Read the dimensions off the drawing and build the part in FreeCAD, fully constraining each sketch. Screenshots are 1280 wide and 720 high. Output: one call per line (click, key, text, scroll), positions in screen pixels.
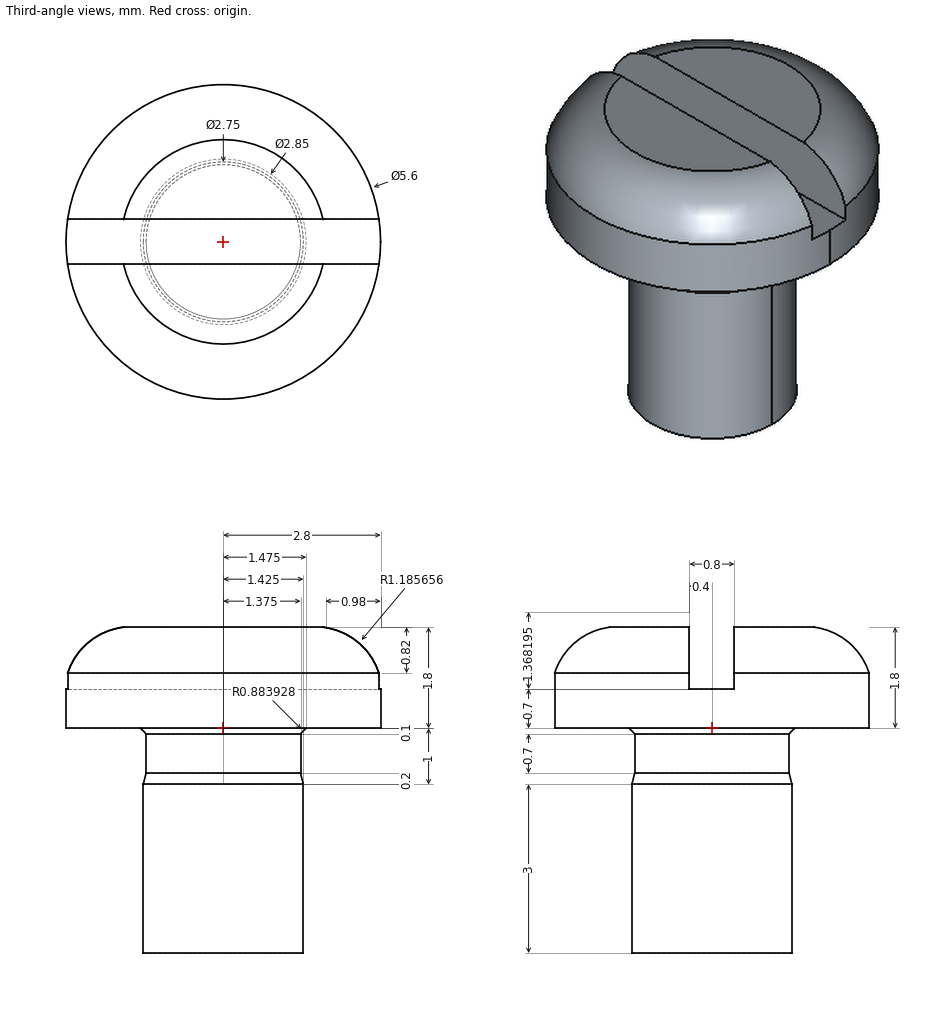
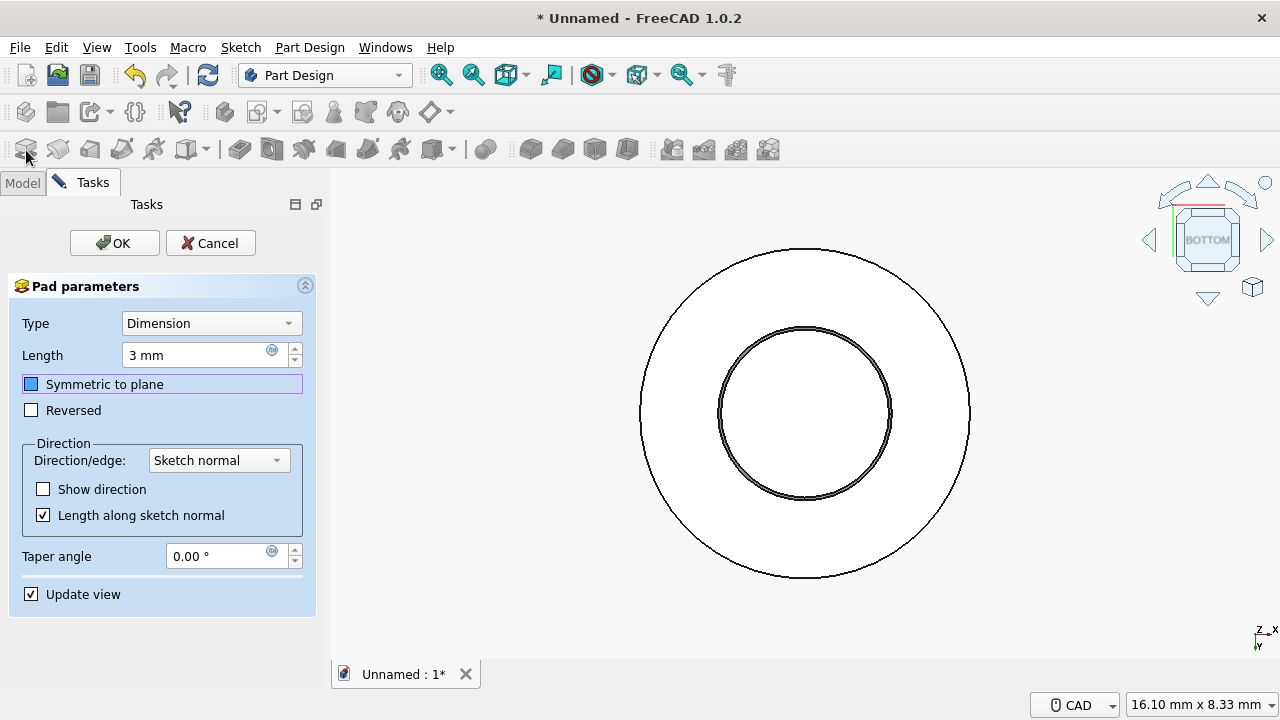
click(115, 243)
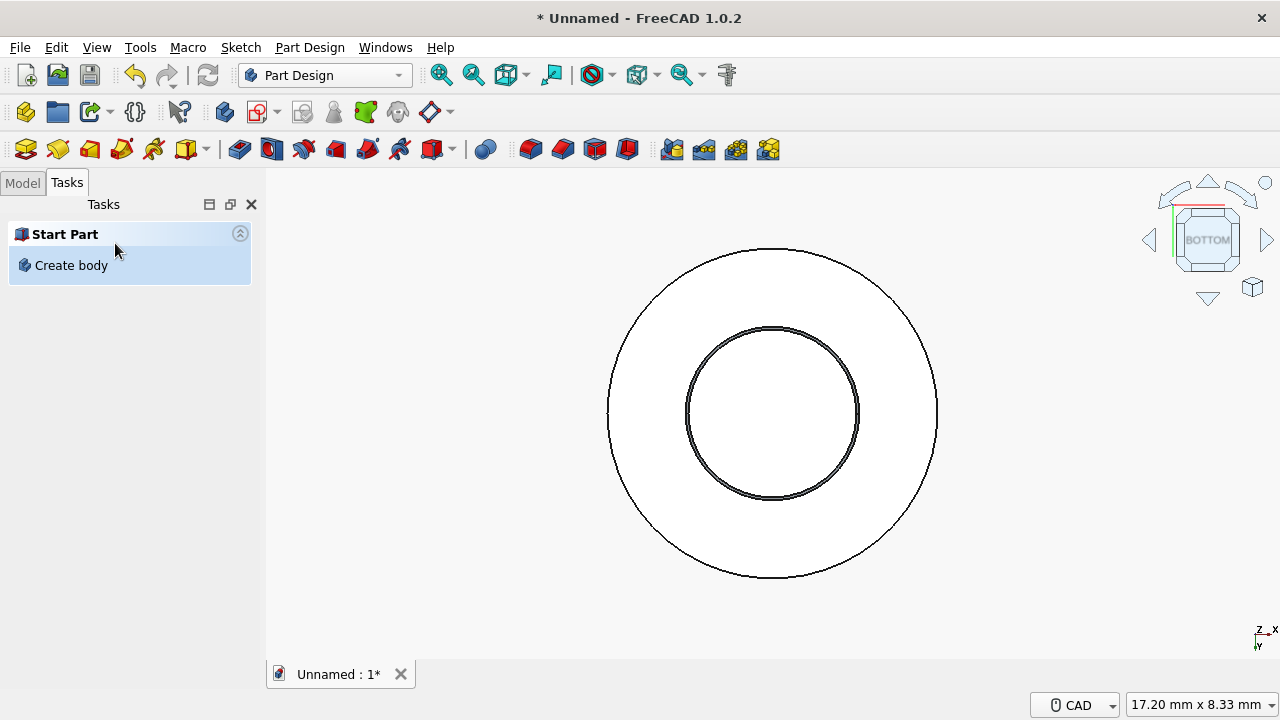
click(258, 112)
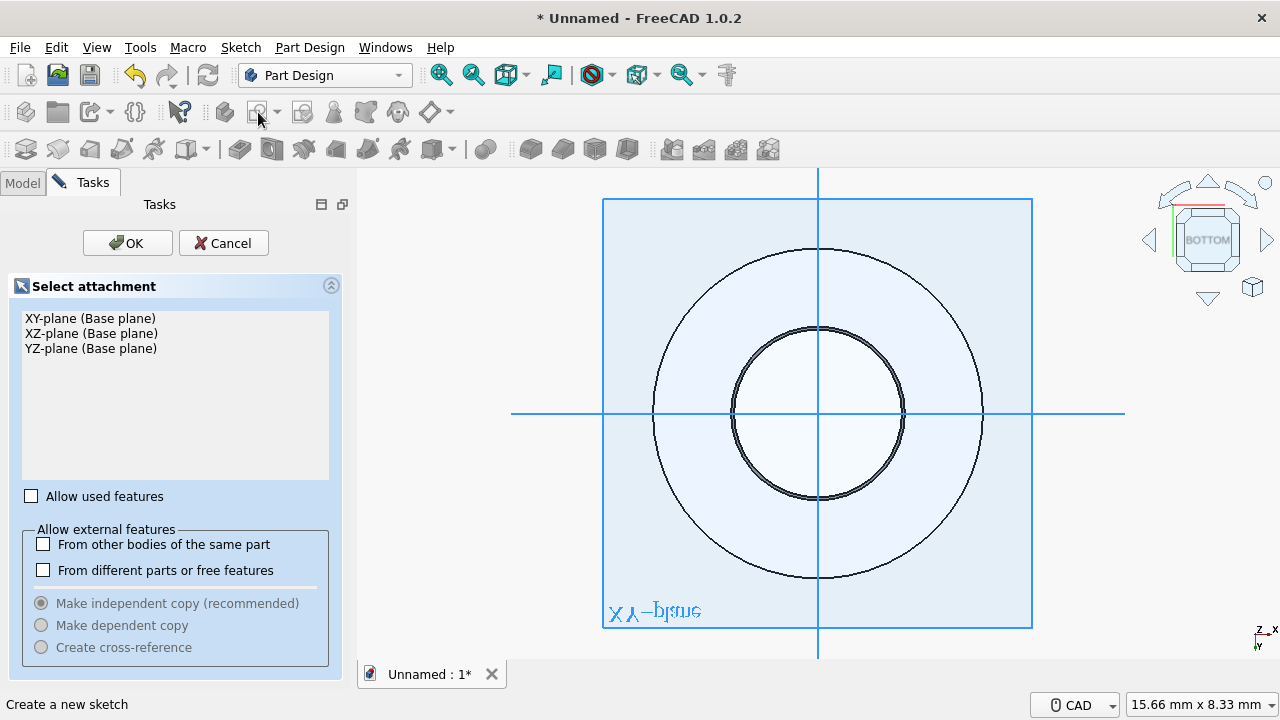
click(82, 334)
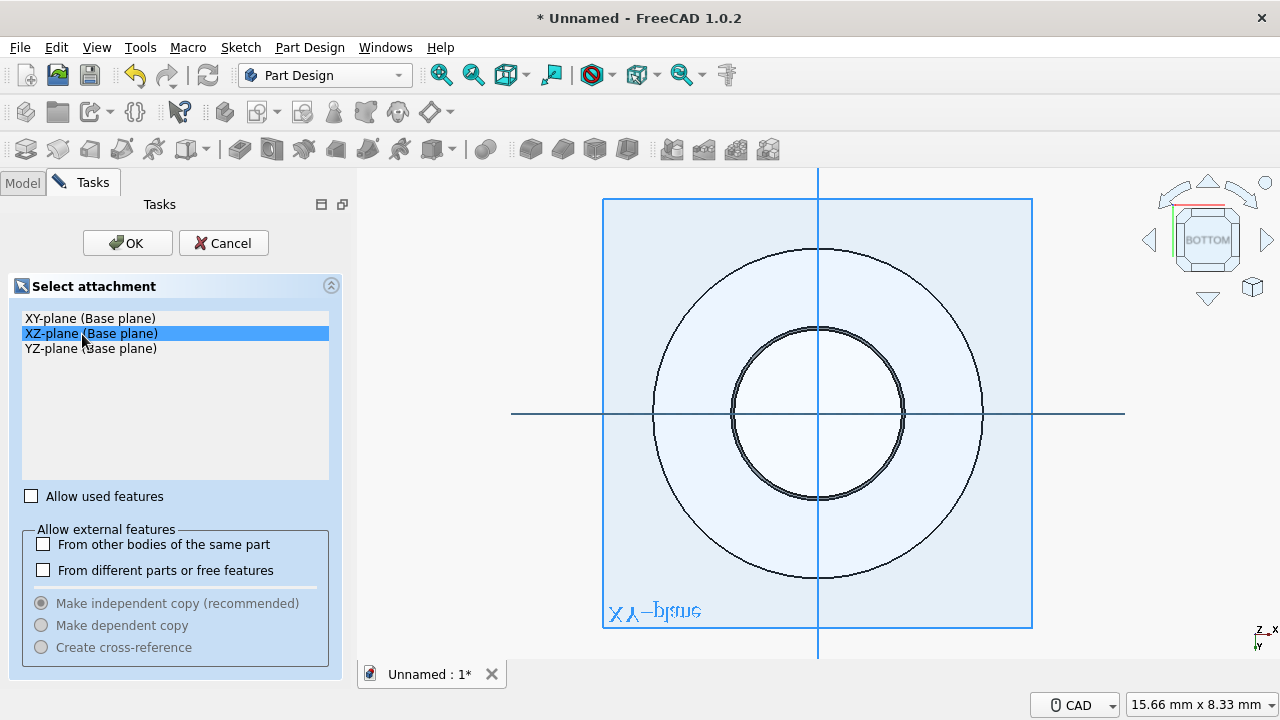
click(128, 243)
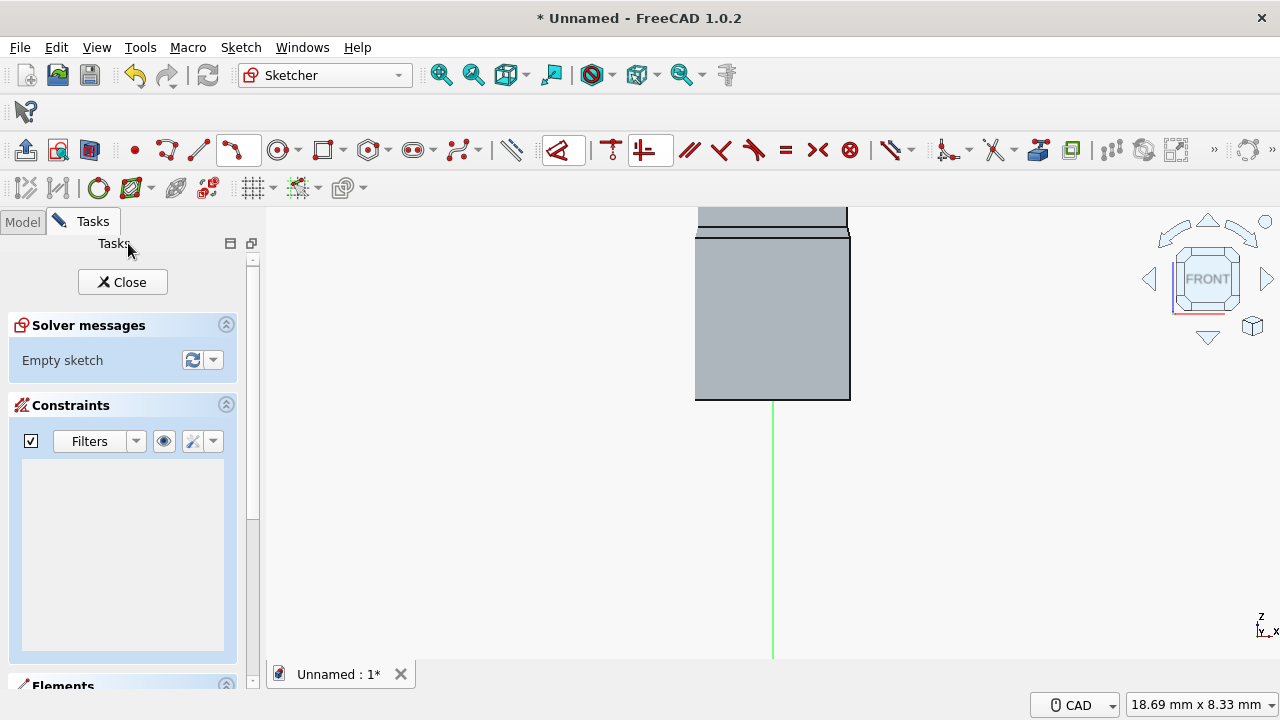
click(90, 150)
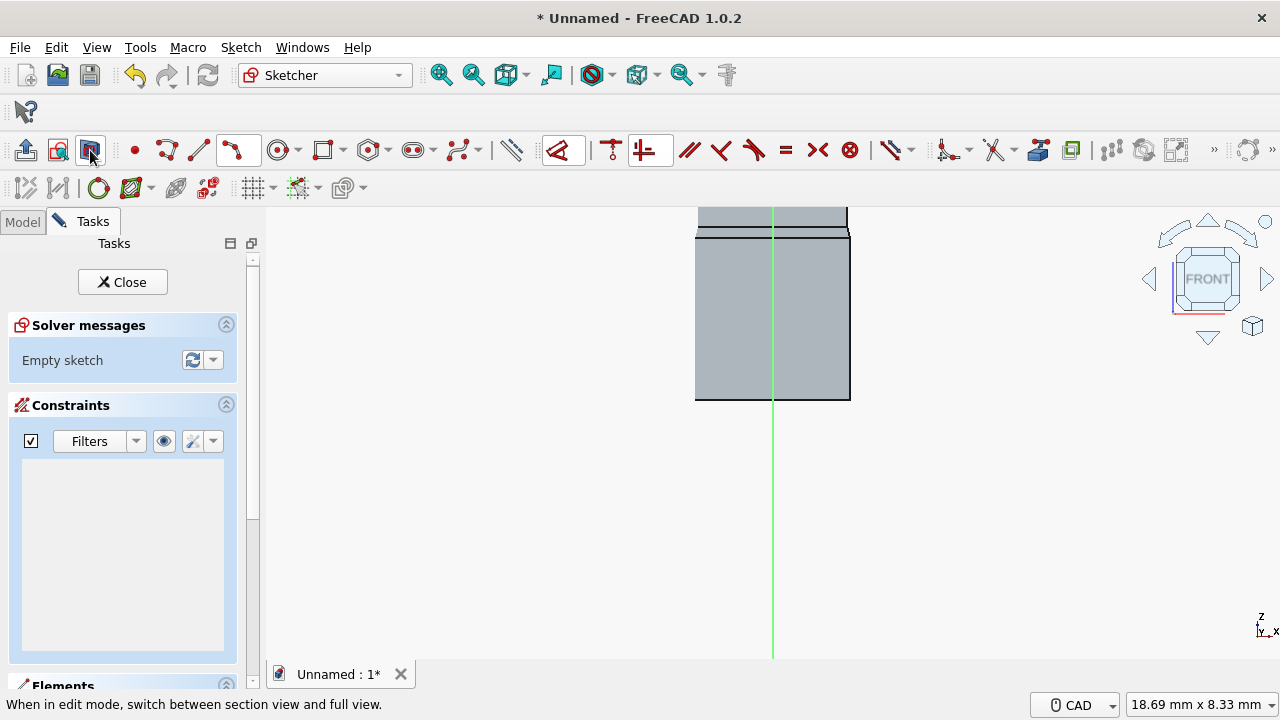
scroll(704, 433, down, 5)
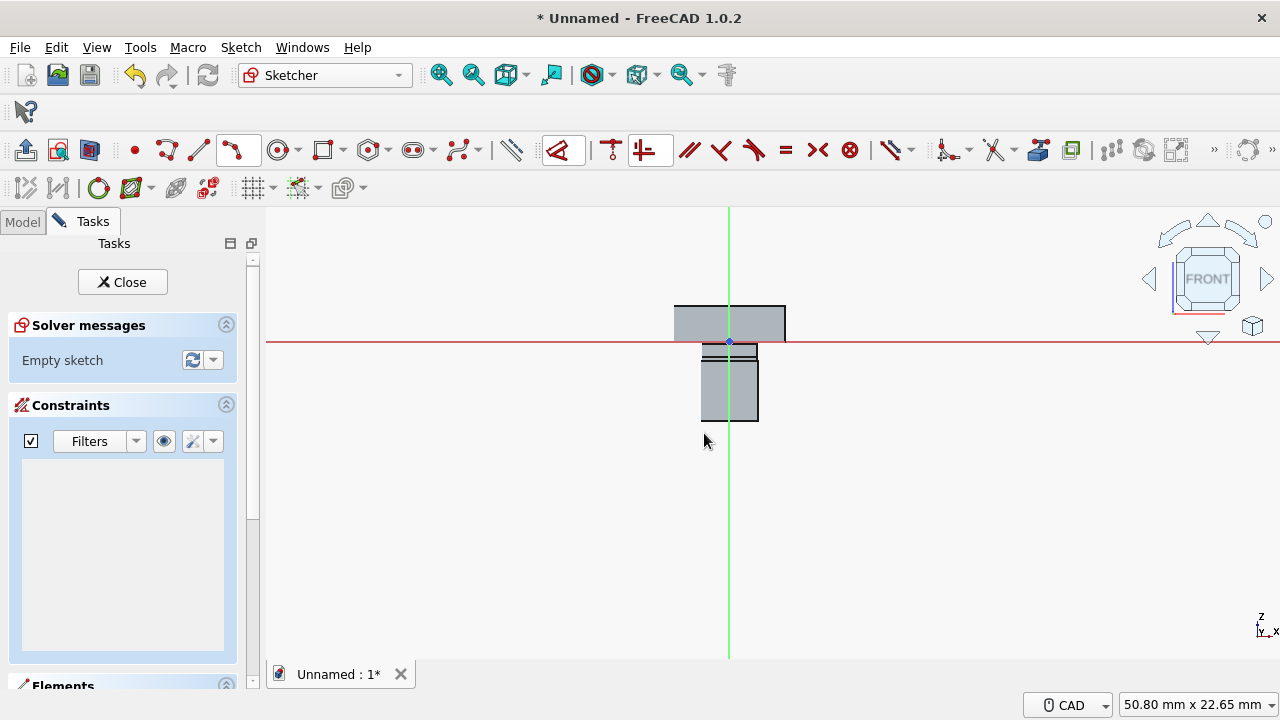
scroll(780, 306, up, 14)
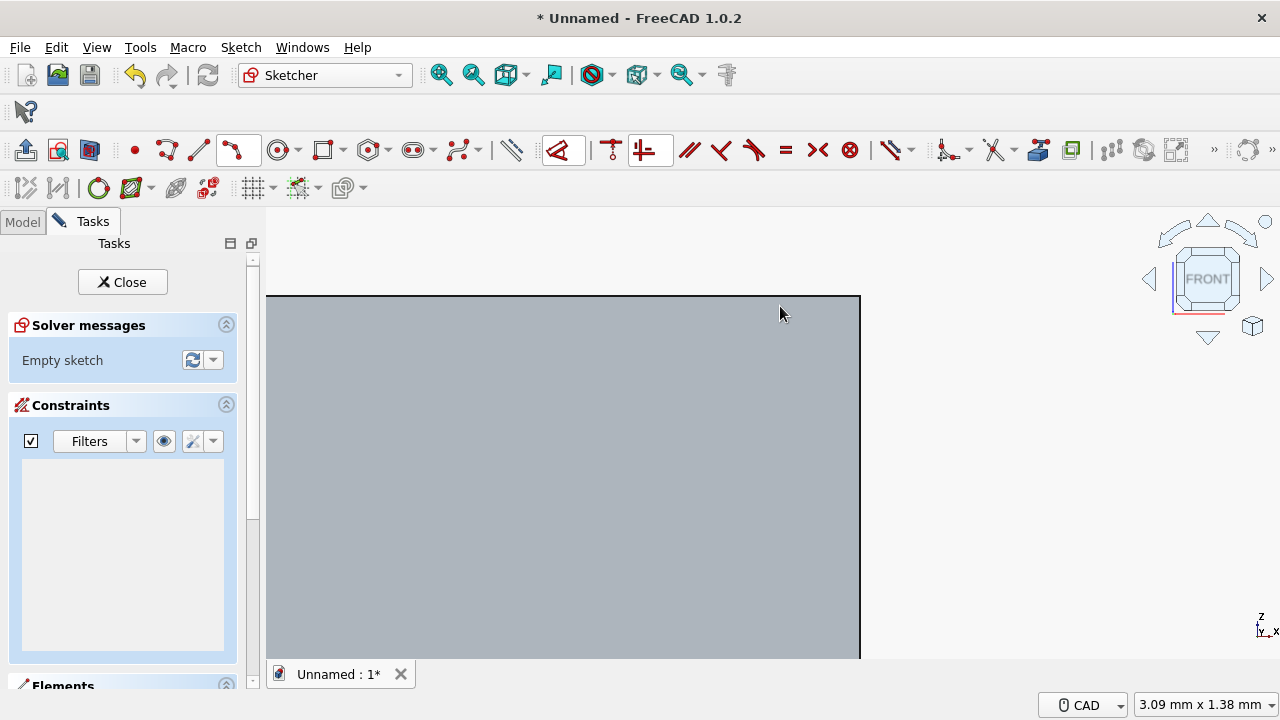
click(168, 150)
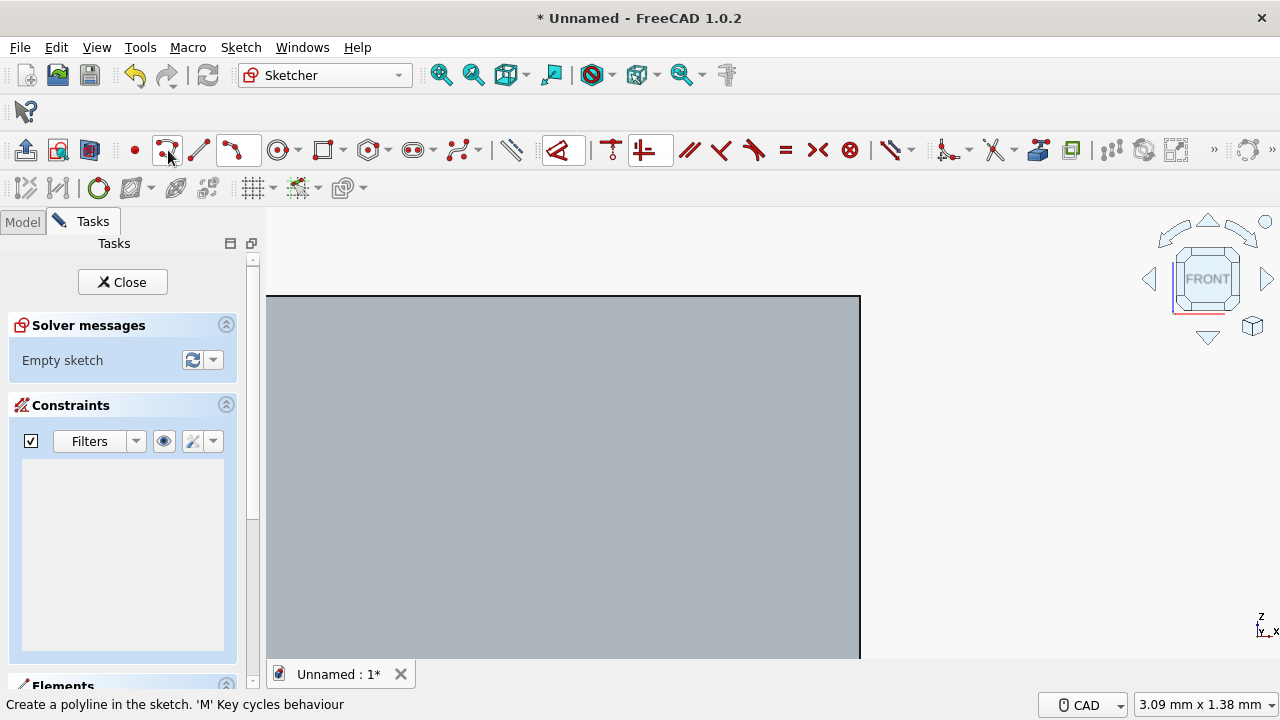
click(539, 296)
click(860, 296)
click(860, 565)
right_click(860, 565)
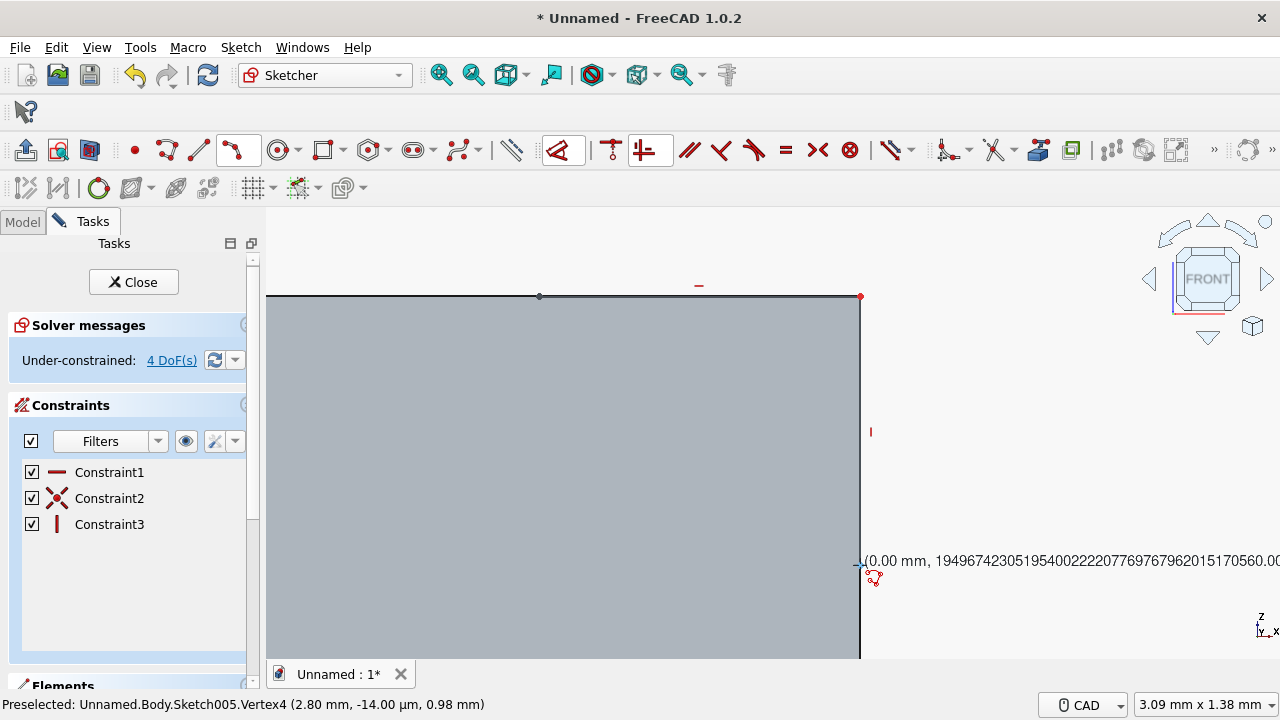
click(232, 150)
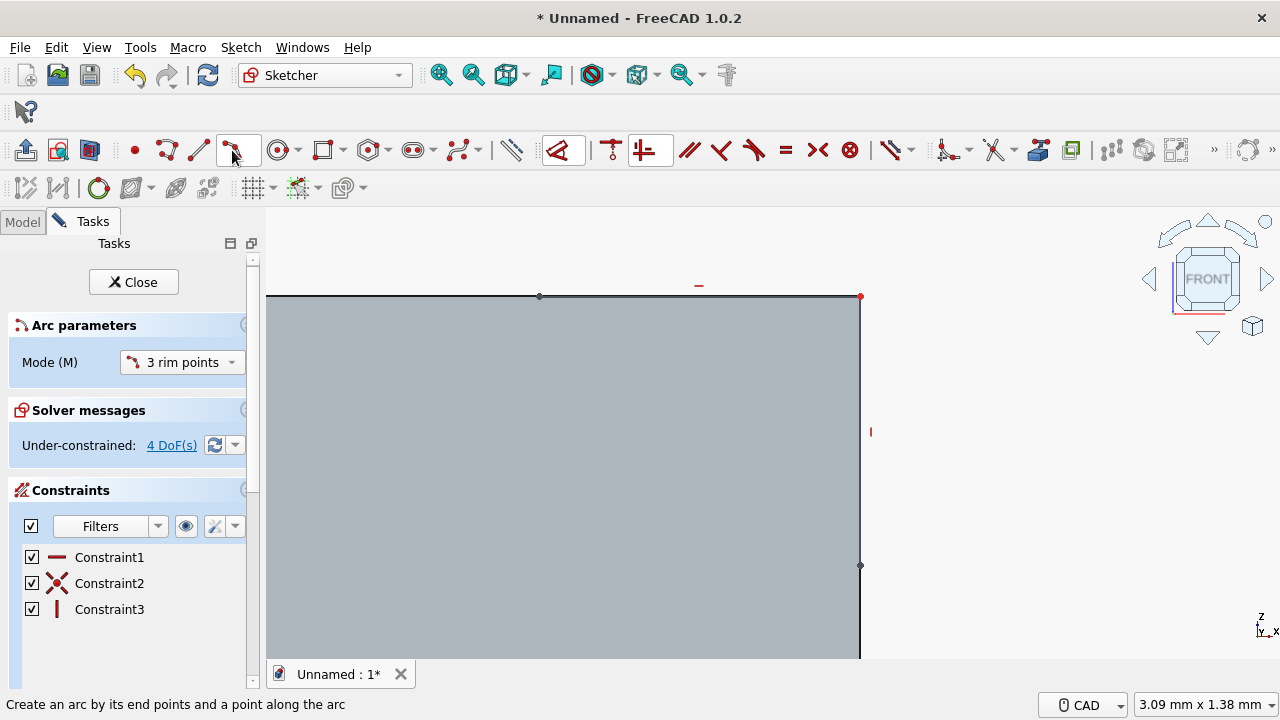
click(860, 566)
click(539, 297)
click(739, 383)
key(Escape)